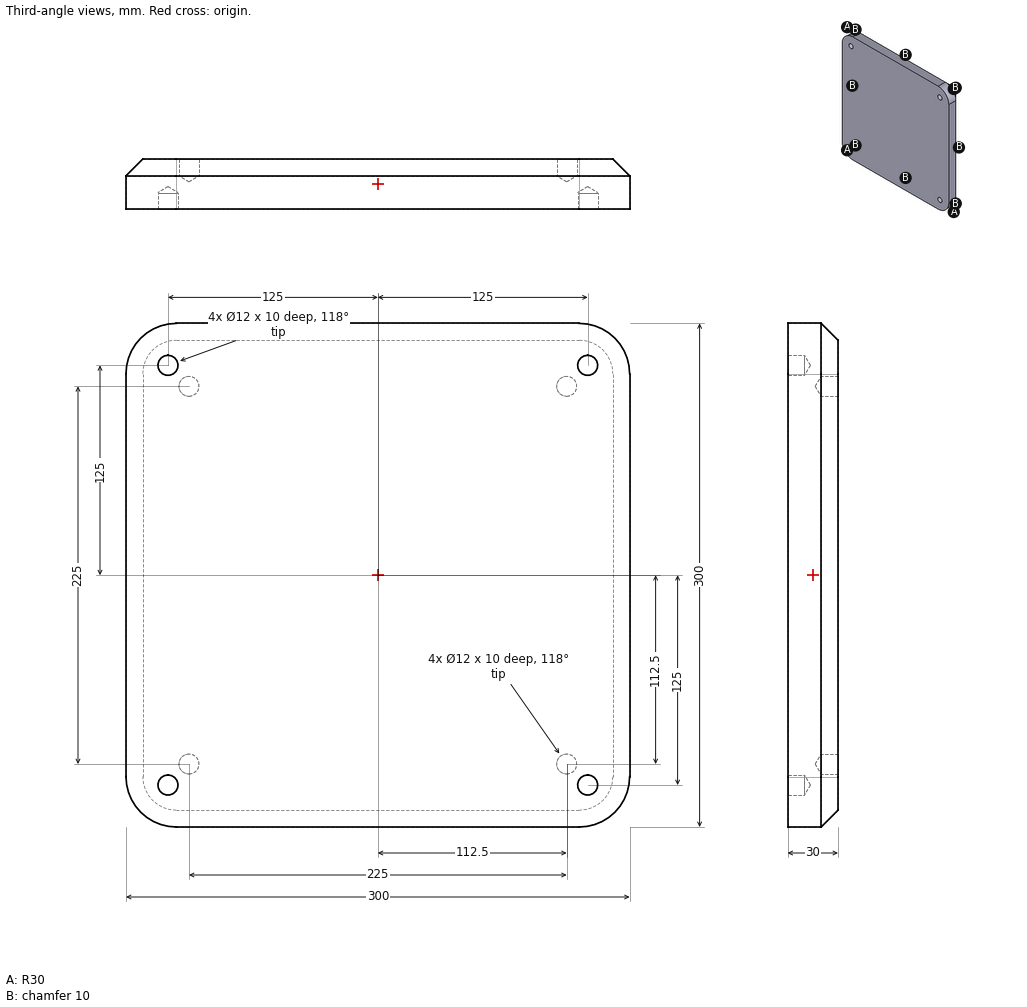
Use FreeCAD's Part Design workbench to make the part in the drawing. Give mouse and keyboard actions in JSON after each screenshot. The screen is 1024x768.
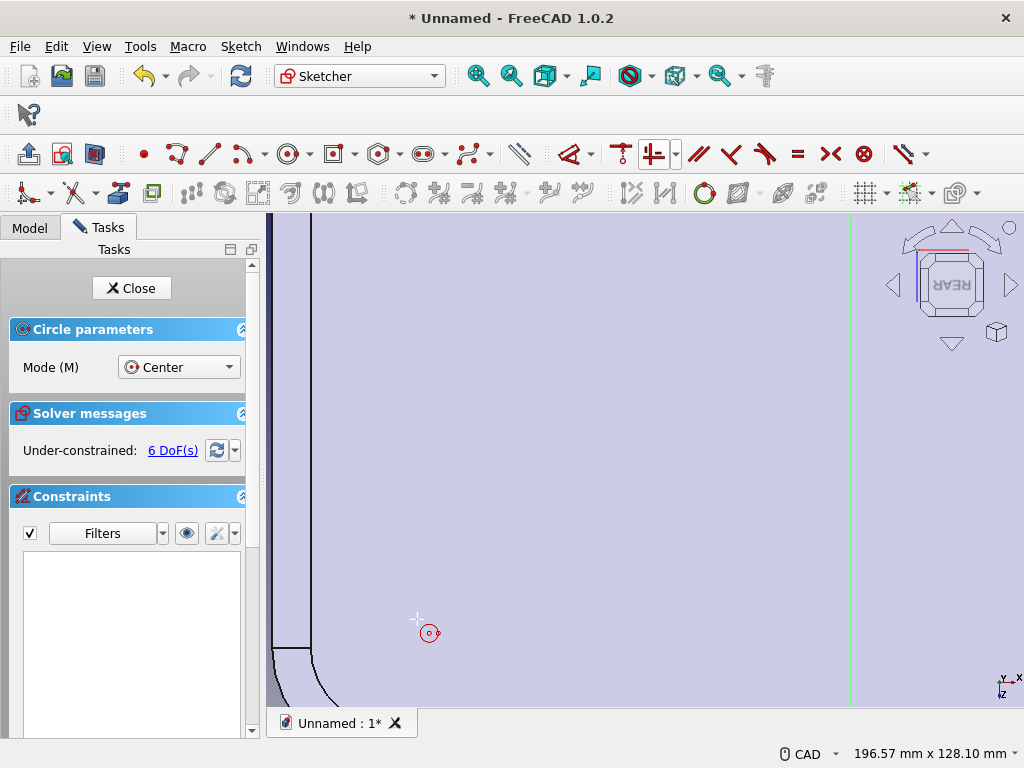
{"action": "left_click", "coordinate": [417, 619]}
{"action": "left_click", "coordinate": [433, 602]}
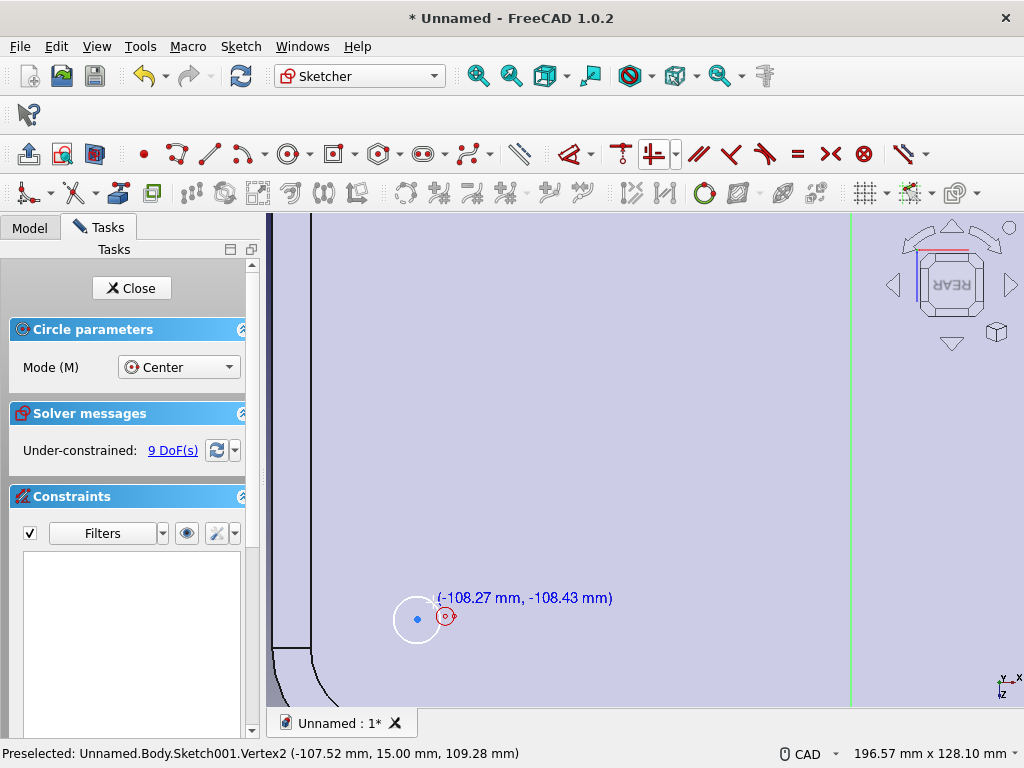
{"action": "scroll", "coordinate": [417, 620], "scroll_direction": "down", "scroll_amount": 5}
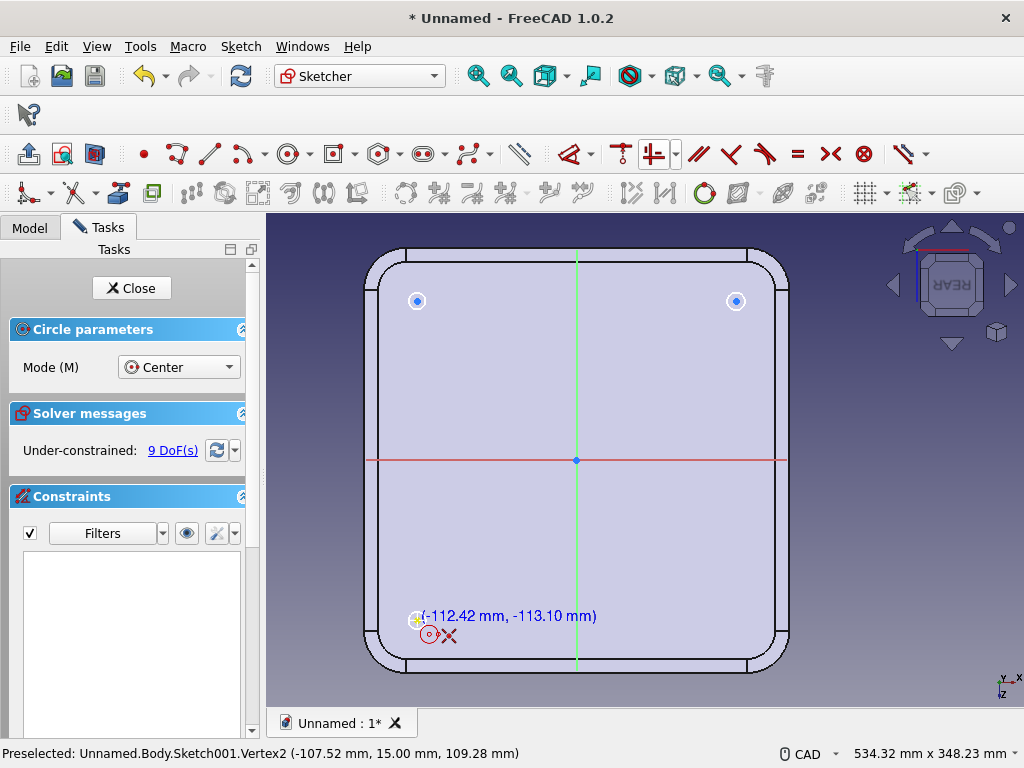
{"action": "scroll", "coordinate": [736, 620], "scroll_direction": "up", "scroll_amount": 5}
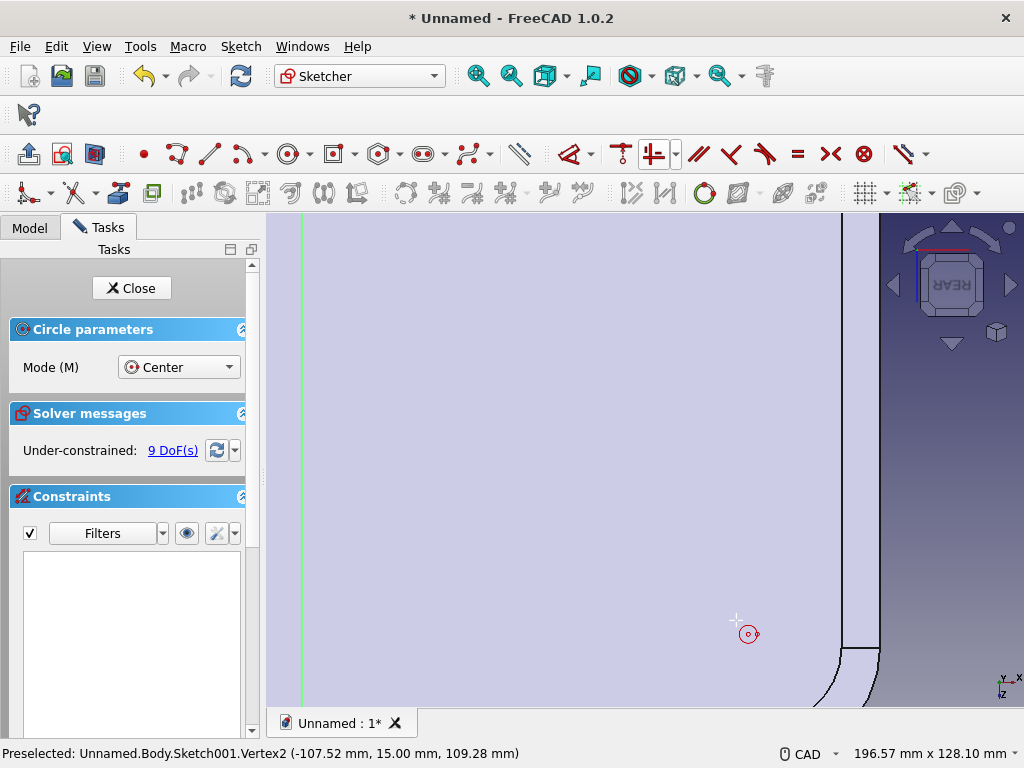
{"action": "left_click", "coordinate": [735, 619]}
{"action": "left_click", "coordinate": [752, 602]}
{"action": "key", "text": "Escape"}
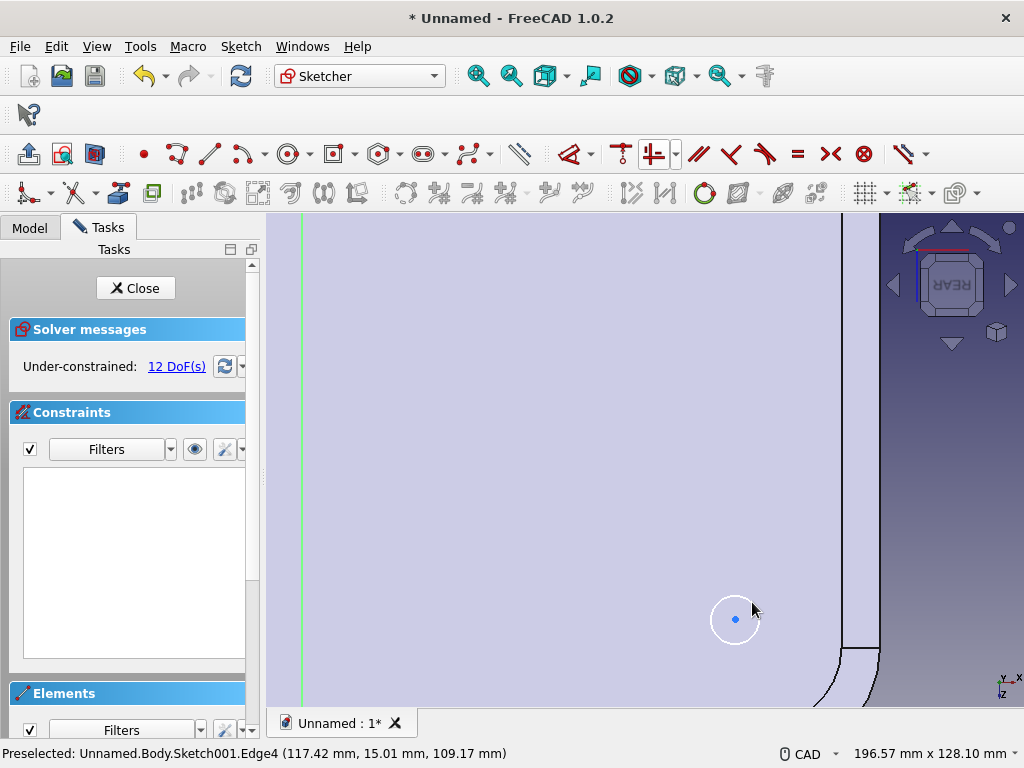
{"action": "scroll", "coordinate": [736, 620], "scroll_direction": "down", "scroll_amount": 5}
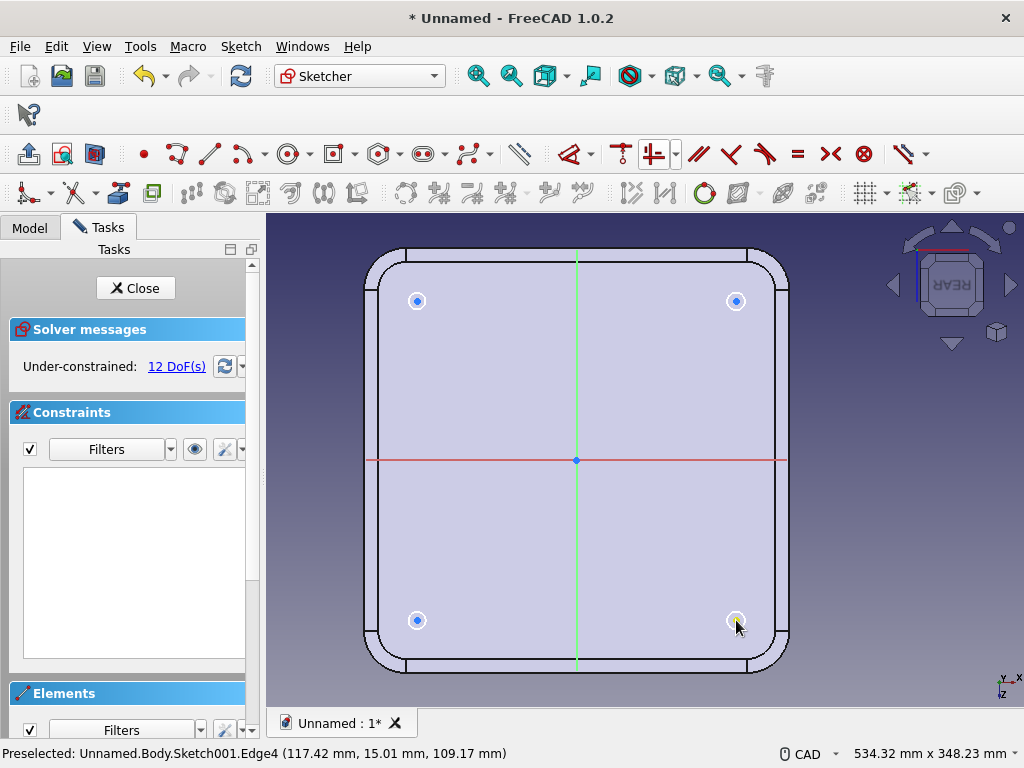
{"action": "scroll", "coordinate": [742, 295], "scroll_direction": "up", "scroll_amount": 3}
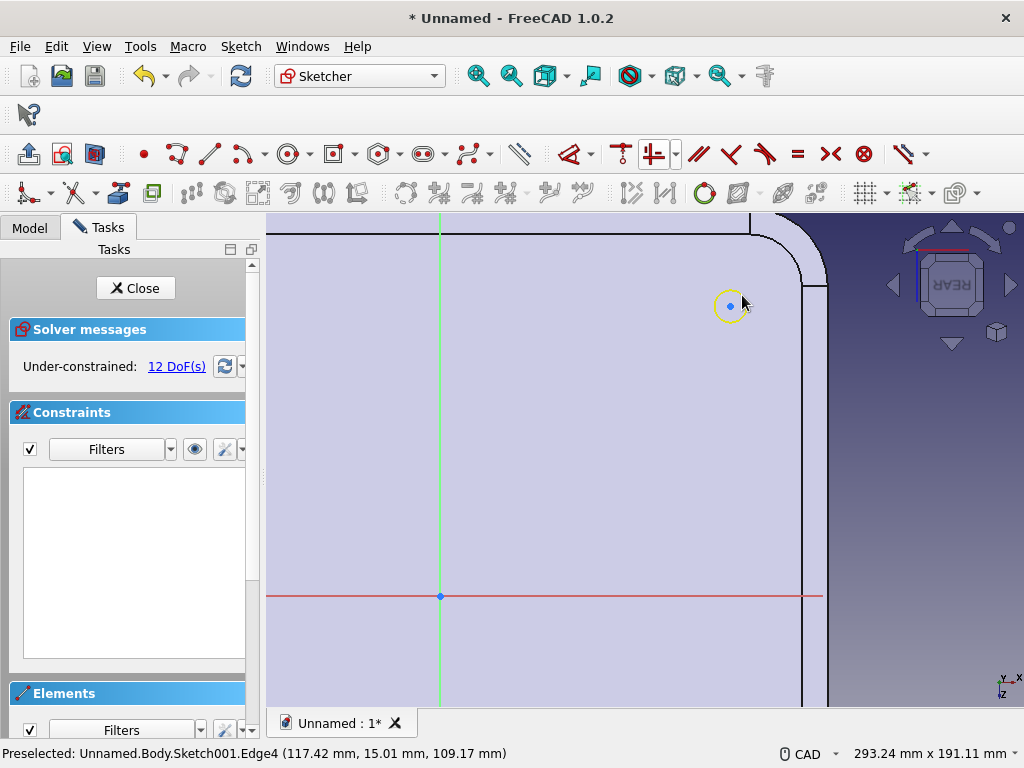
{"action": "left_click", "coordinate": [742, 295]}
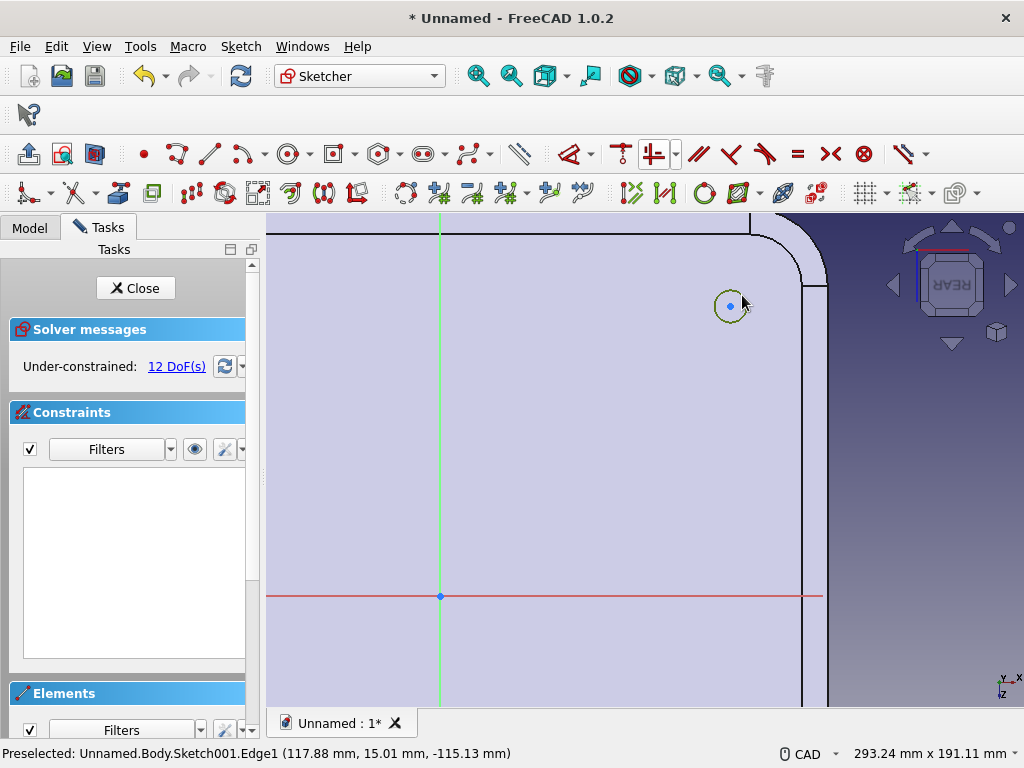
{"action": "scroll", "coordinate": [742, 294], "scroll_direction": "down", "scroll_amount": 3}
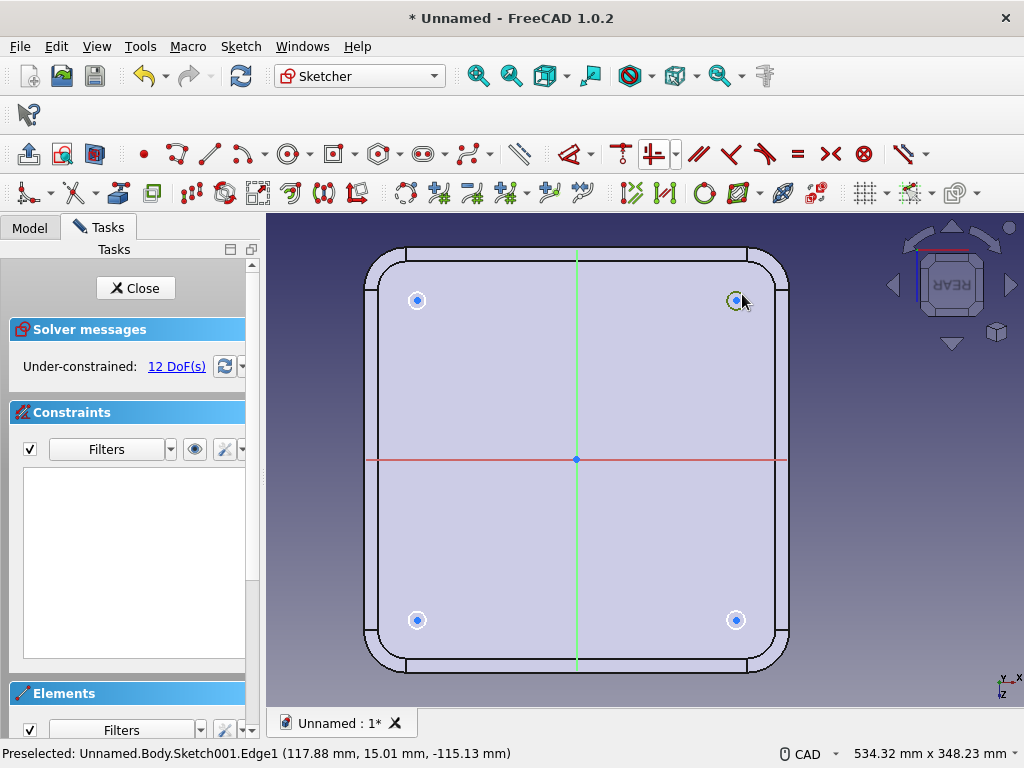
{"action": "scroll", "coordinate": [423, 295], "scroll_direction": "up", "scroll_amount": 3}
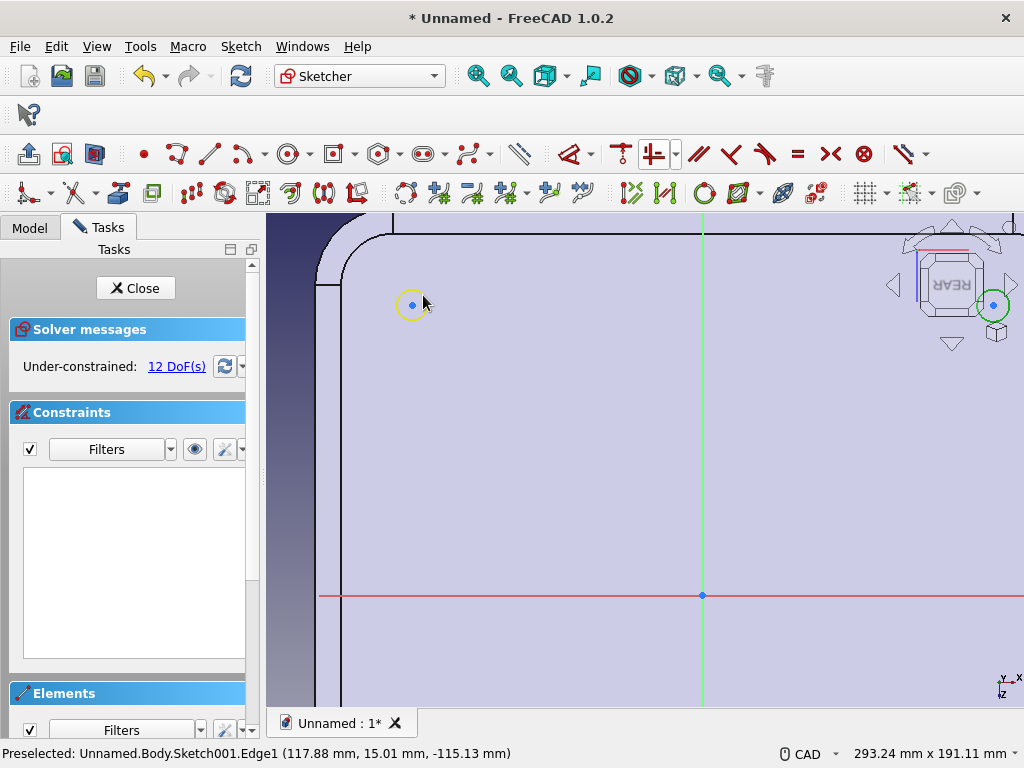
{"action": "left_click", "coordinate": [423, 294]}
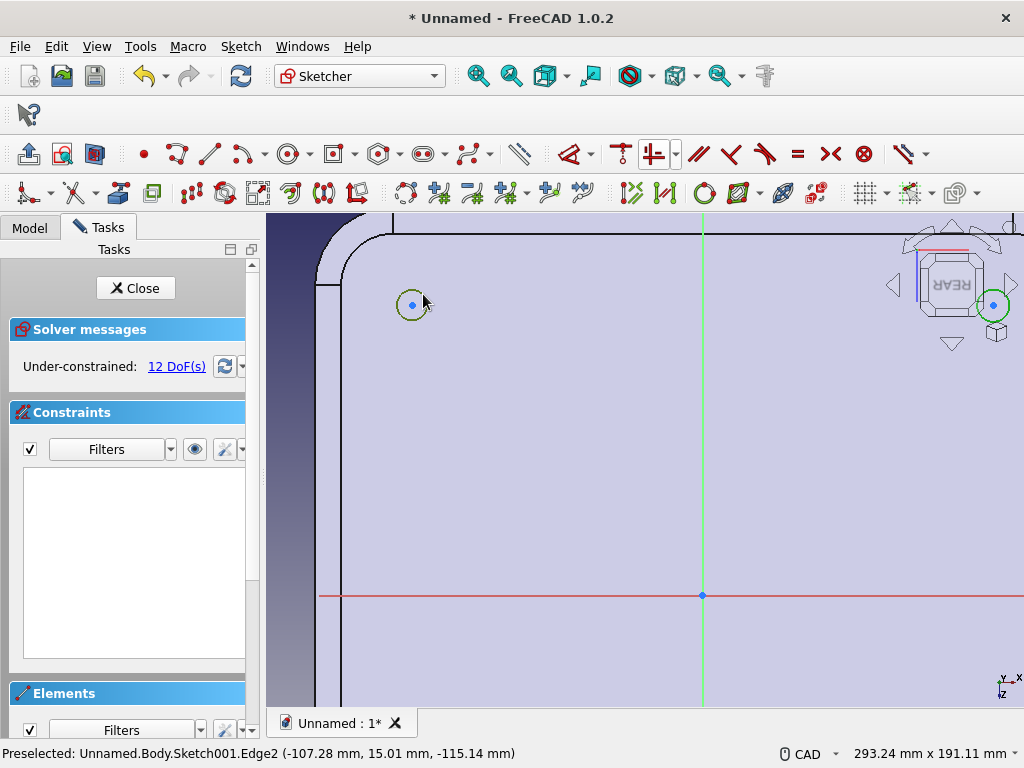
{"action": "scroll", "coordinate": [423, 295], "scroll_direction": "down", "scroll_amount": 3}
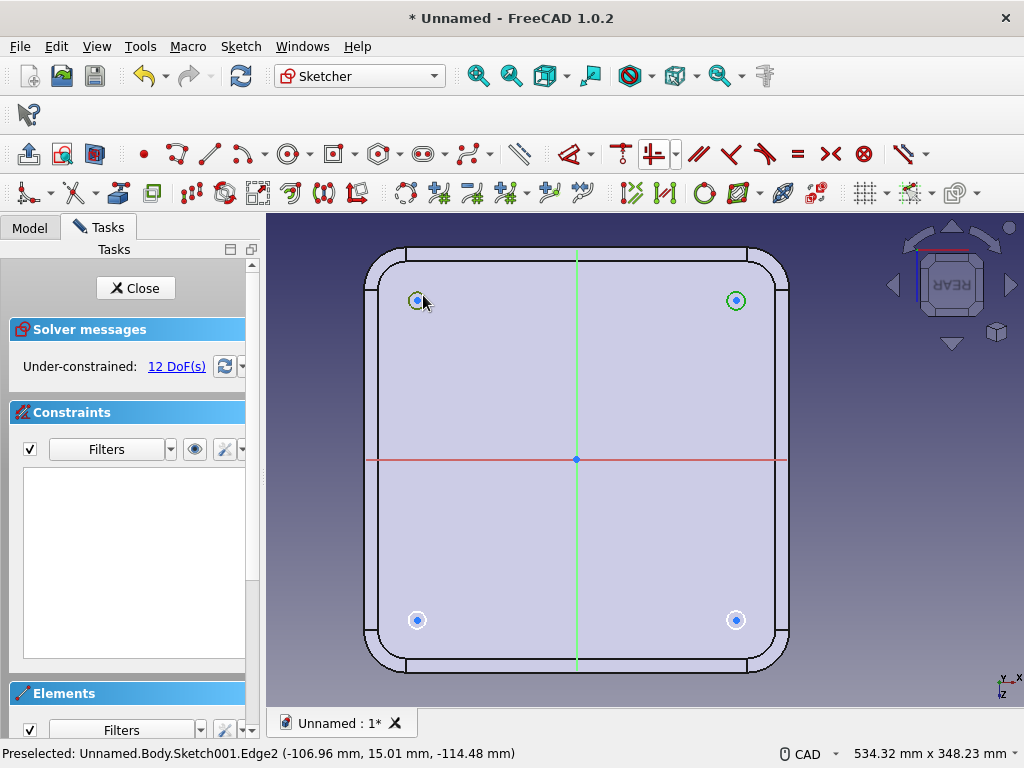
{"action": "scroll", "coordinate": [423, 614], "scroll_direction": "up", "scroll_amount": 3}